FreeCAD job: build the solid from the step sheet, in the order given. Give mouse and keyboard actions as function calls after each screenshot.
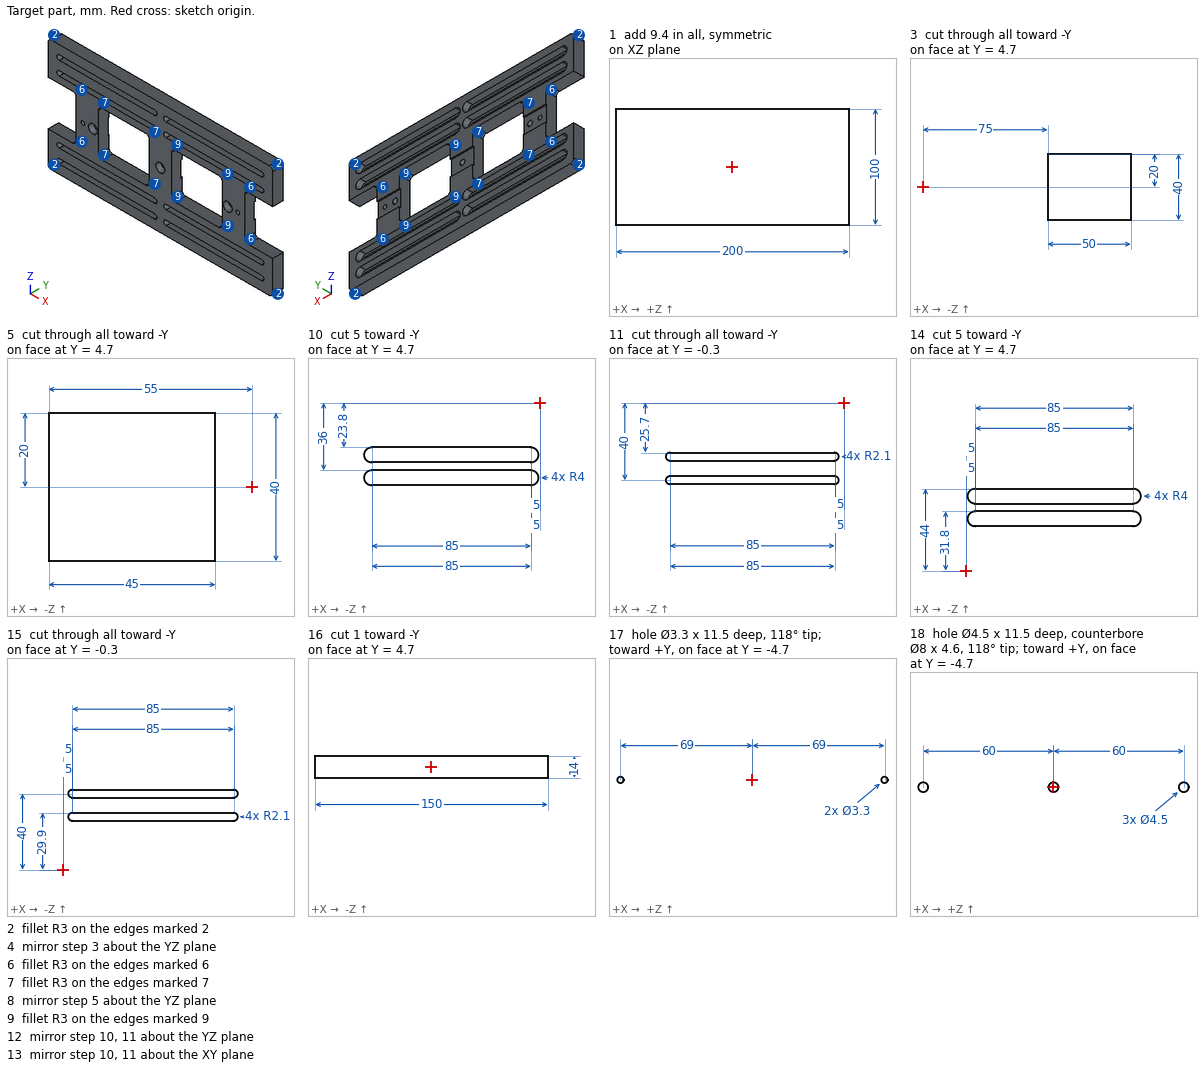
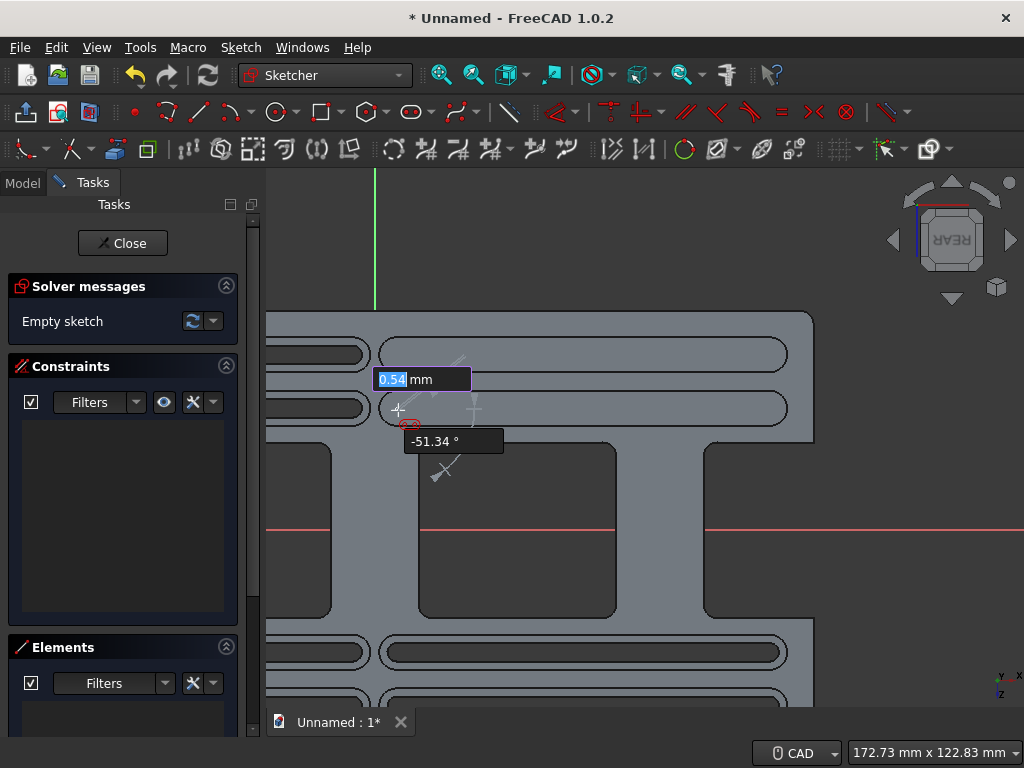
click(770, 408)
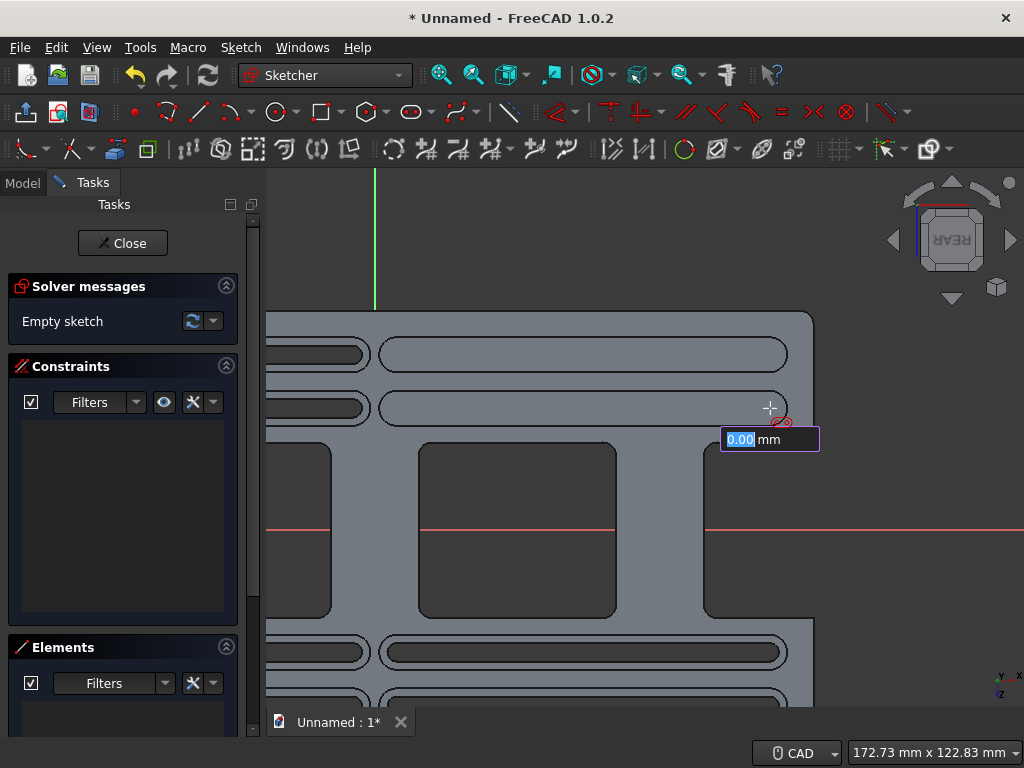
scroll(583, 418, up, 3)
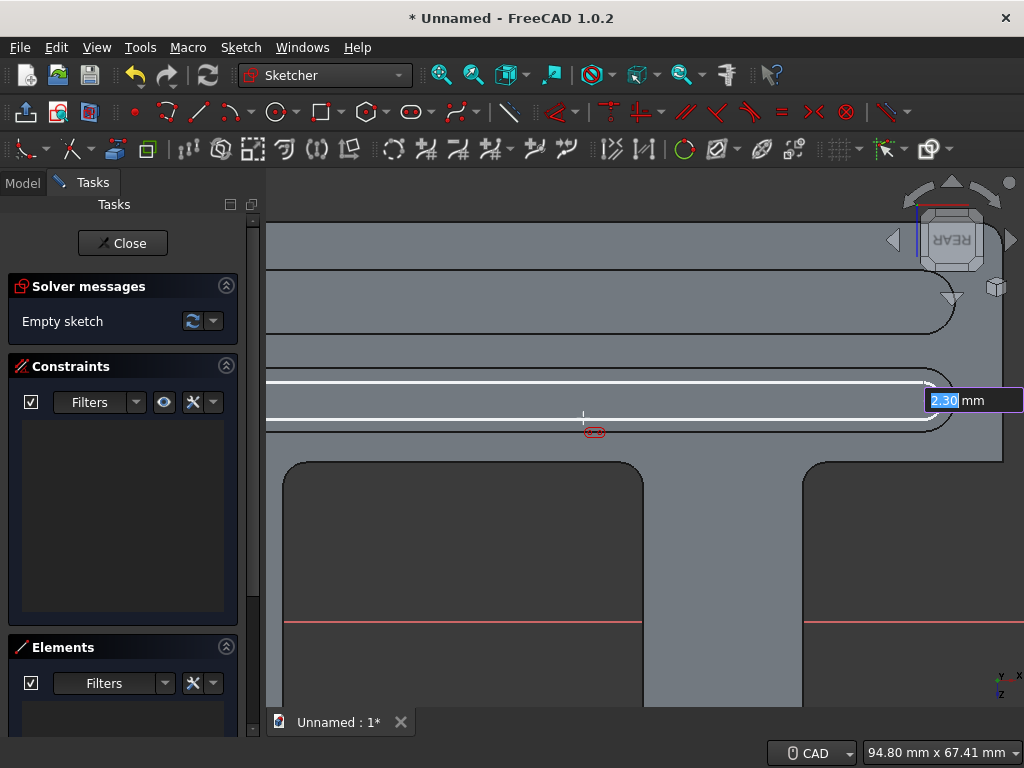
click(583, 417)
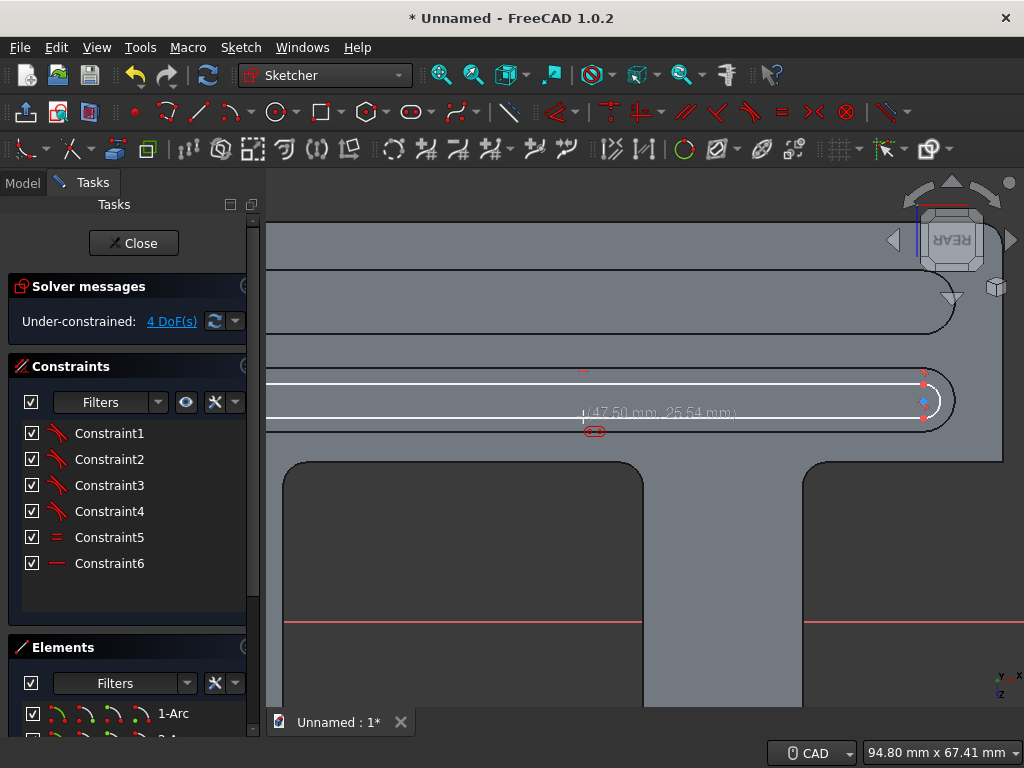
scroll(583, 418, down, 3)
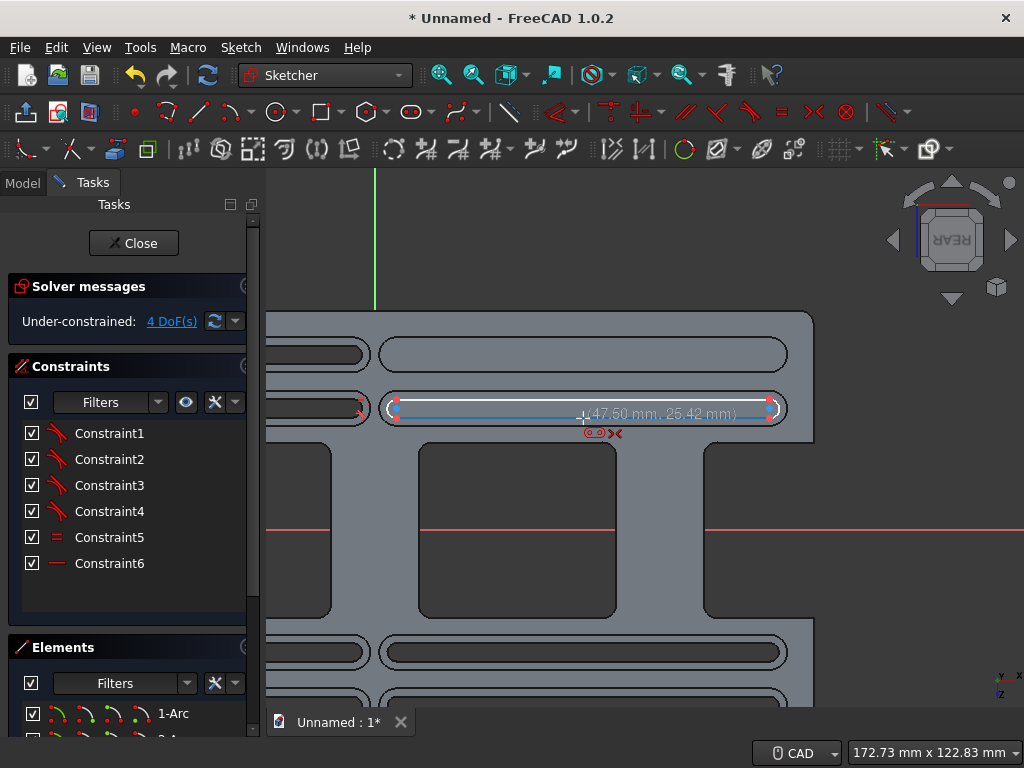
scroll(397, 355, up, 5)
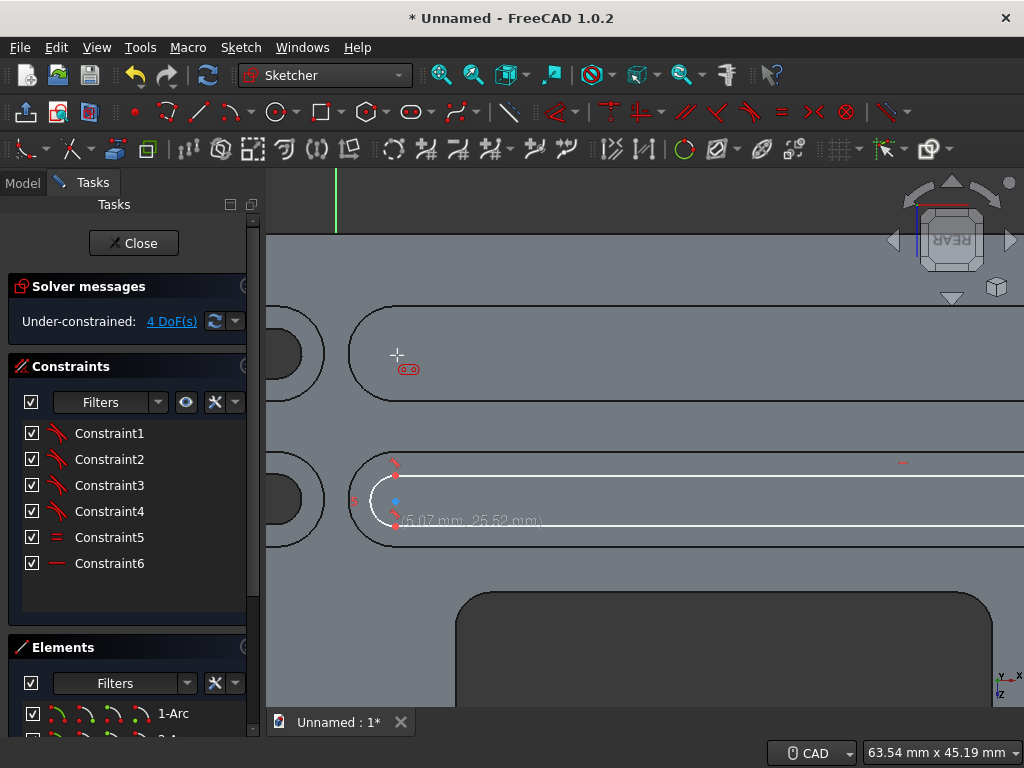
click(396, 354)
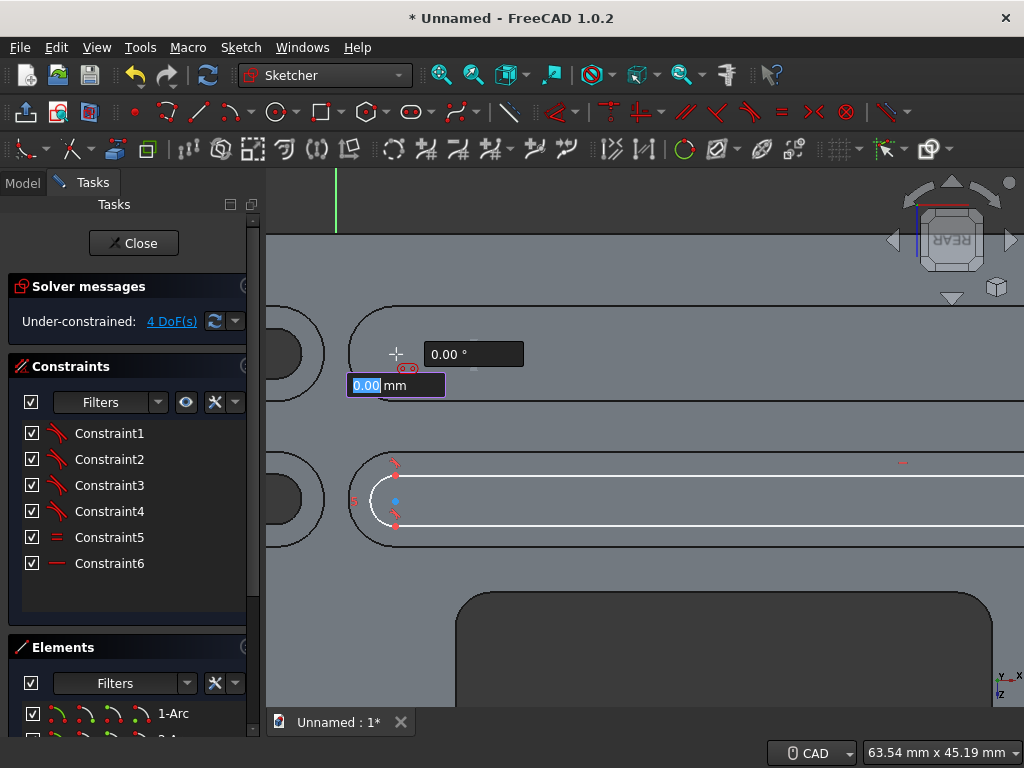
scroll(397, 355, down, 5)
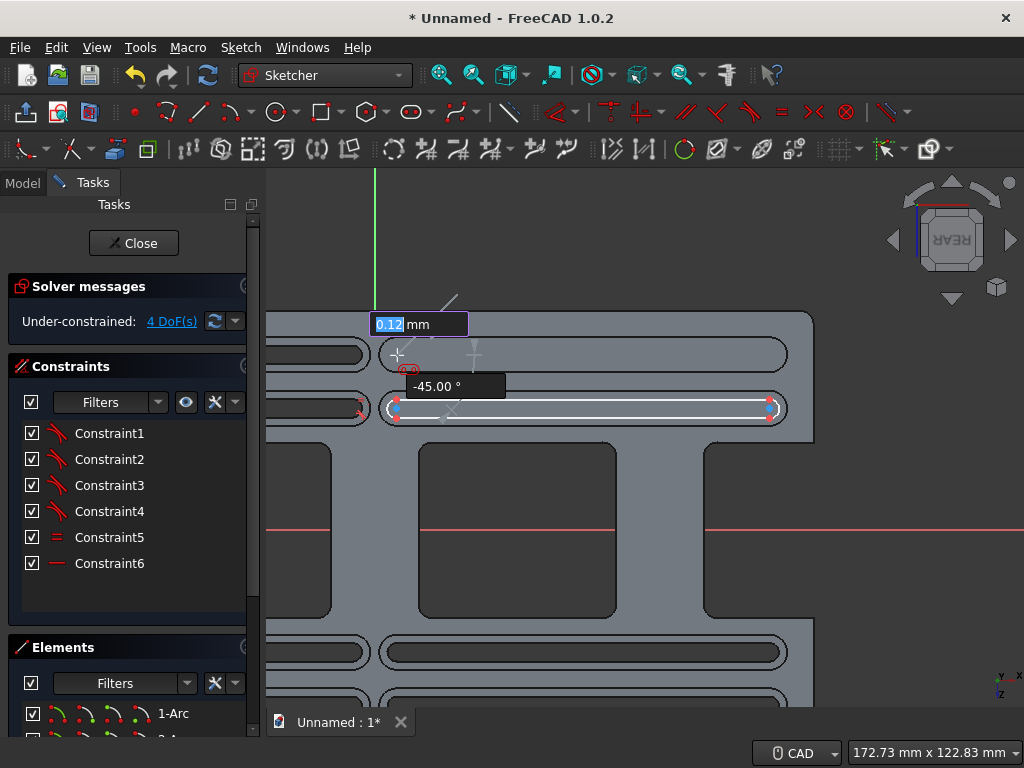
click(770, 355)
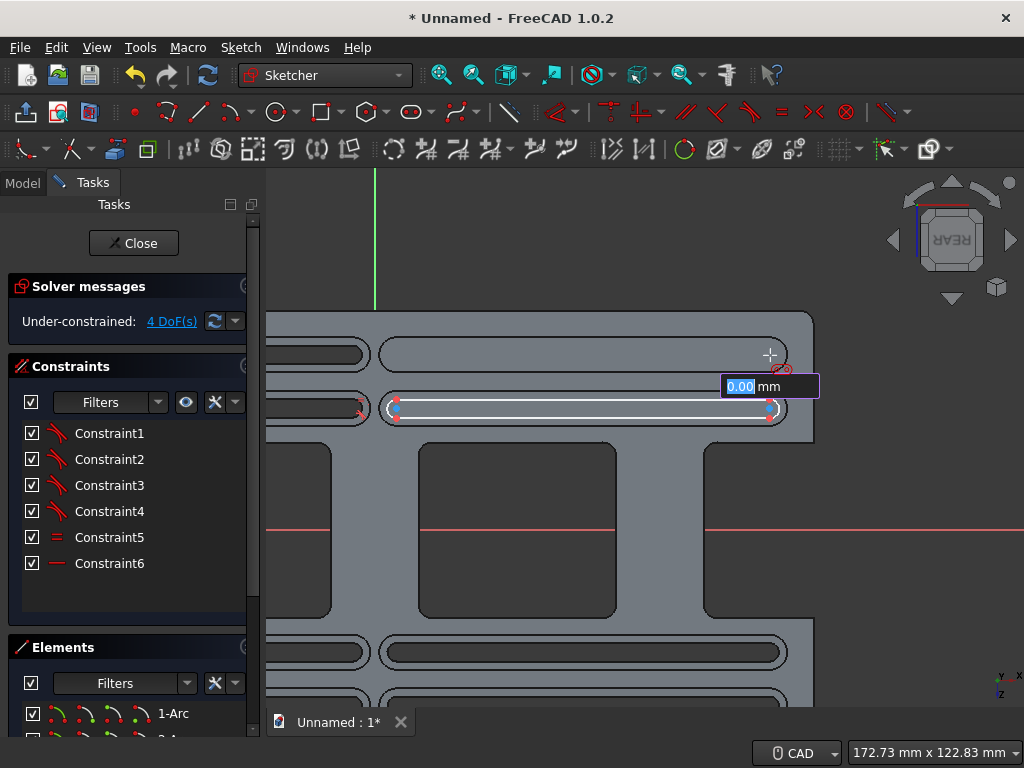
scroll(583, 364, up, 3)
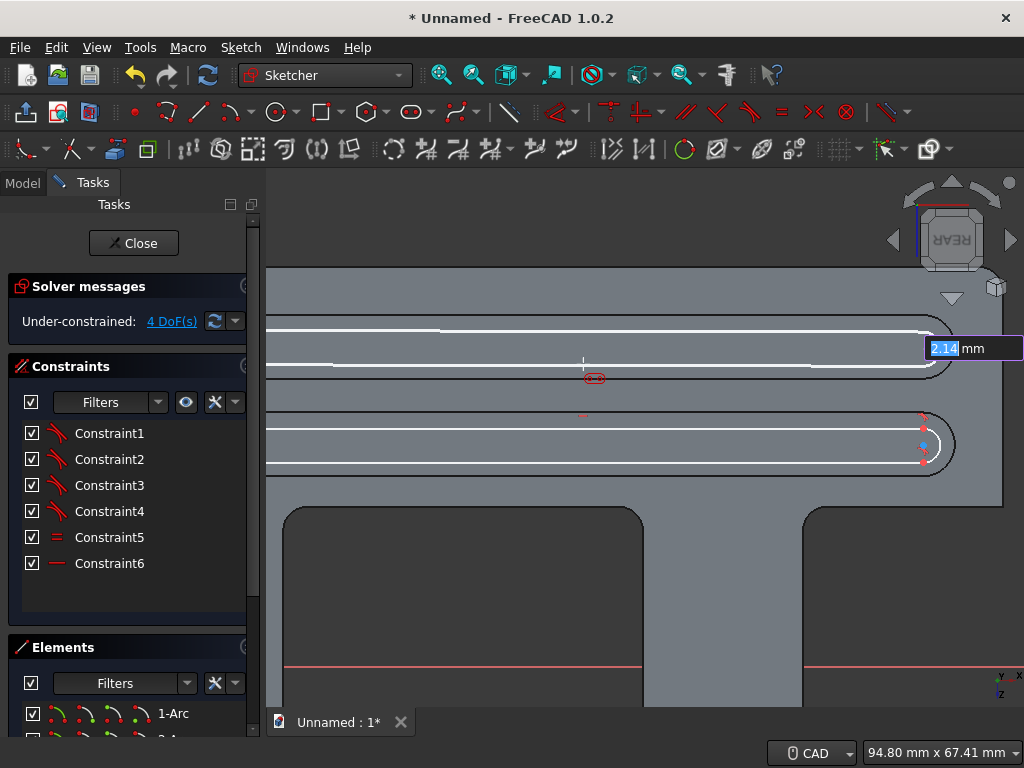
click(583, 364)
key(Escape)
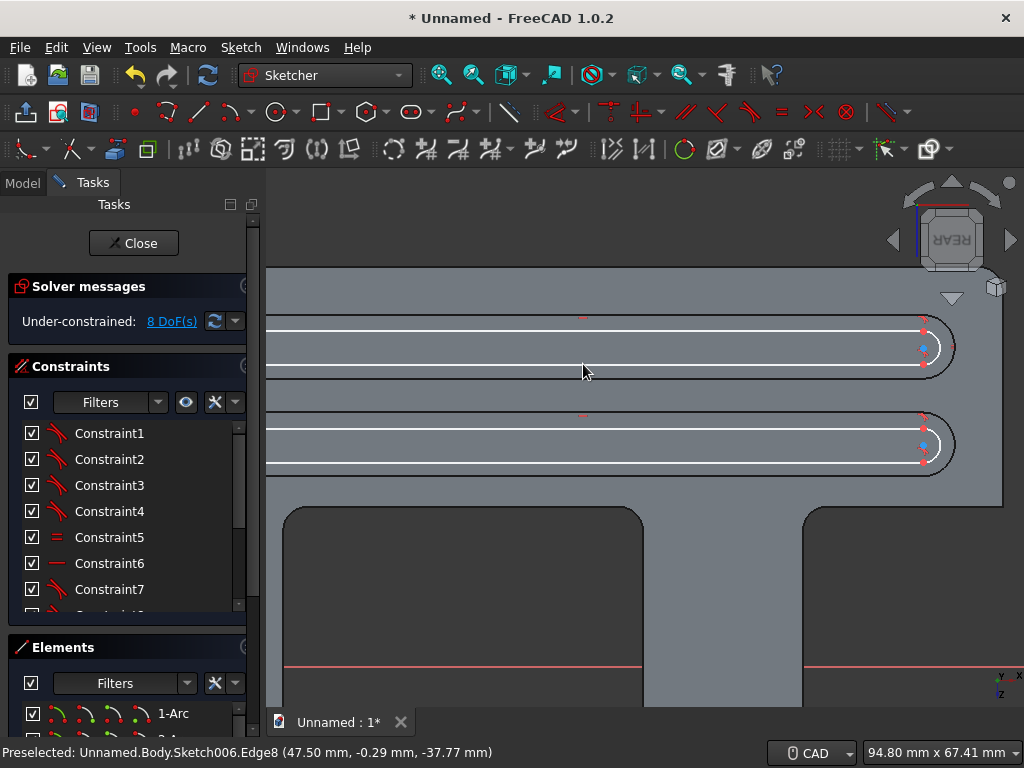
scroll(583, 363, down, 3)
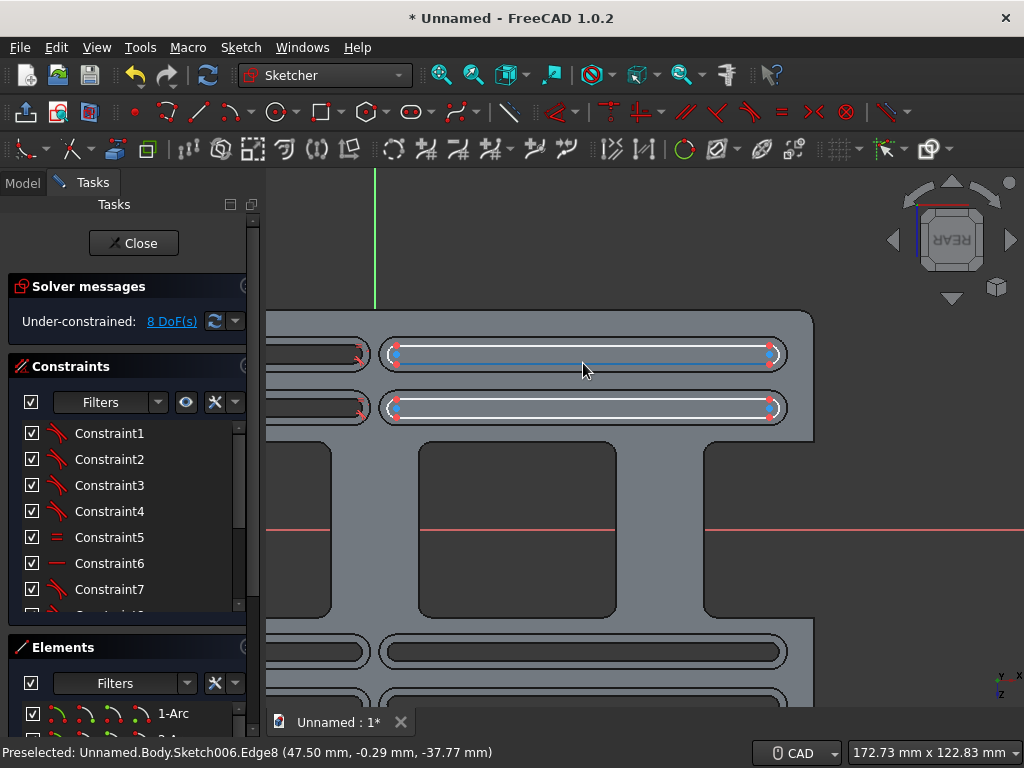
scroll(389, 403, up, 3)